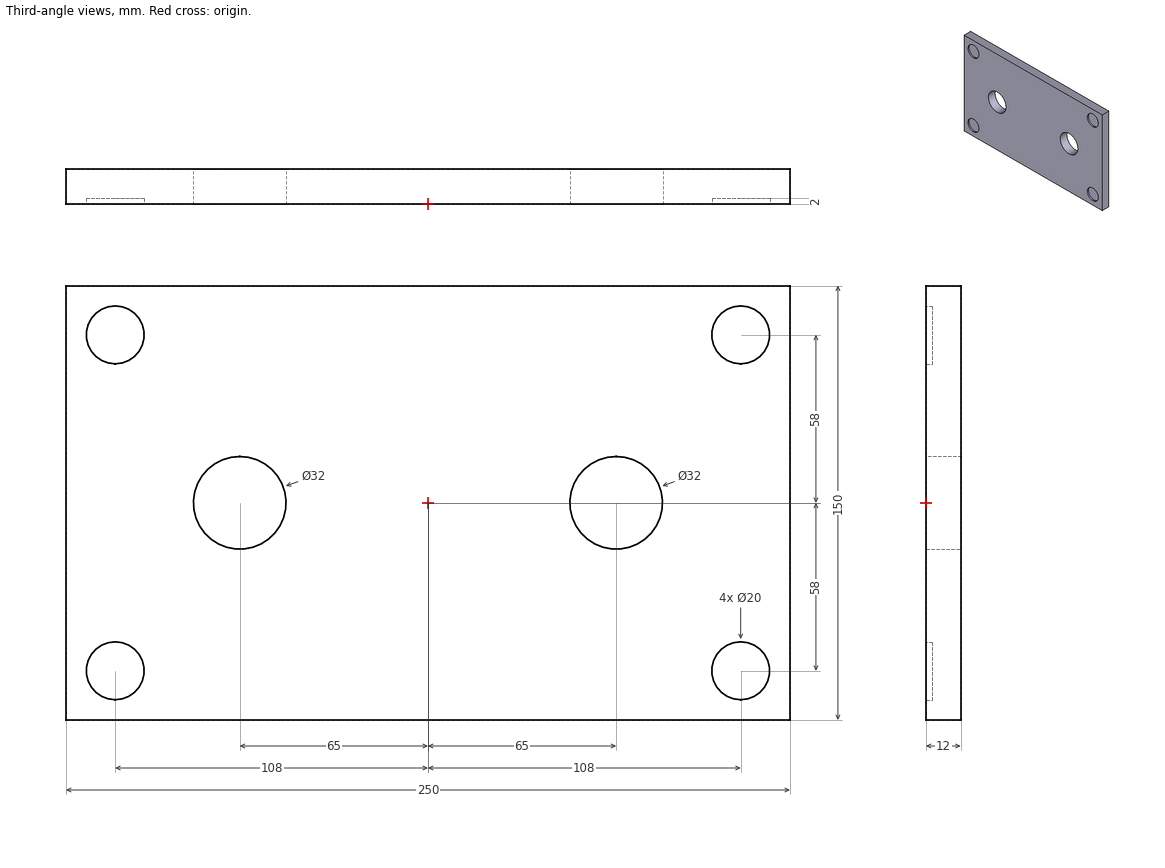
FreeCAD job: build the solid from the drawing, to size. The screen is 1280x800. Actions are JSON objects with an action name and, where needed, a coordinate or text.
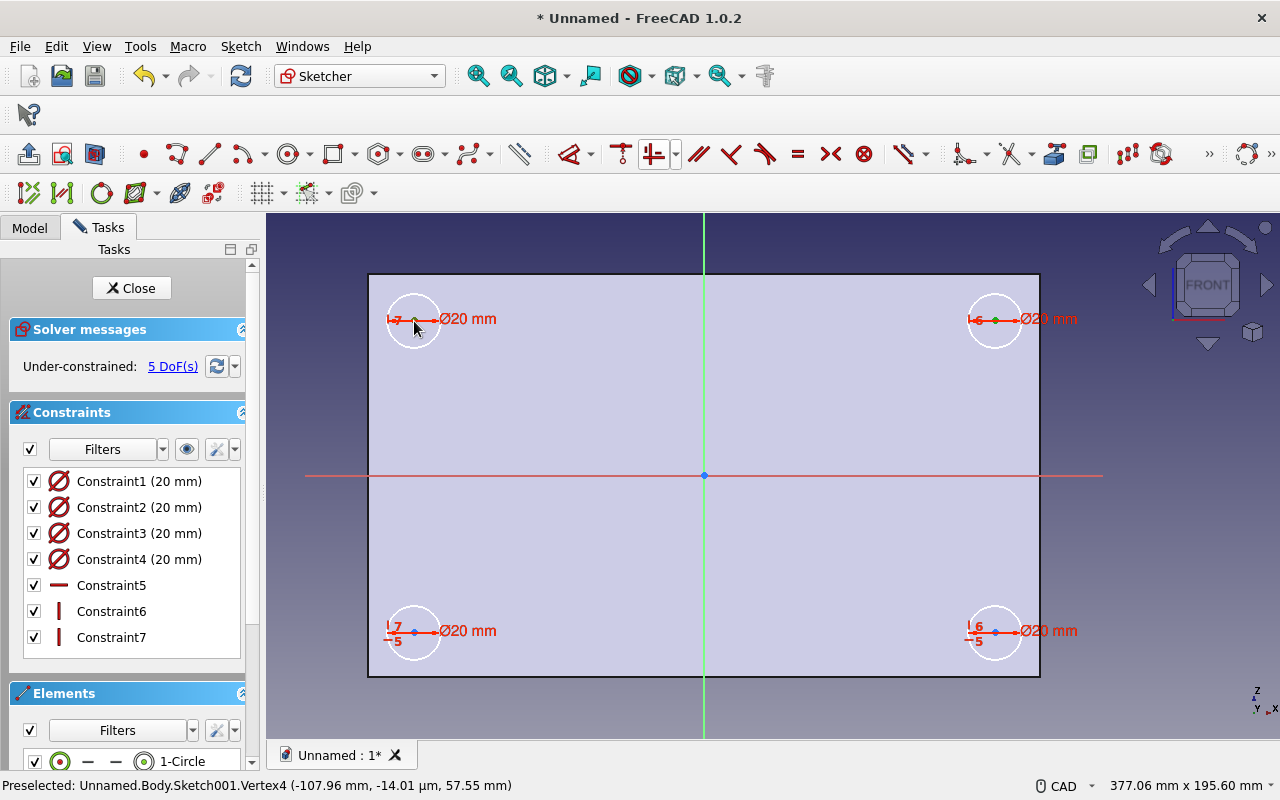
{"action": "left_click", "coordinate": [676, 154]}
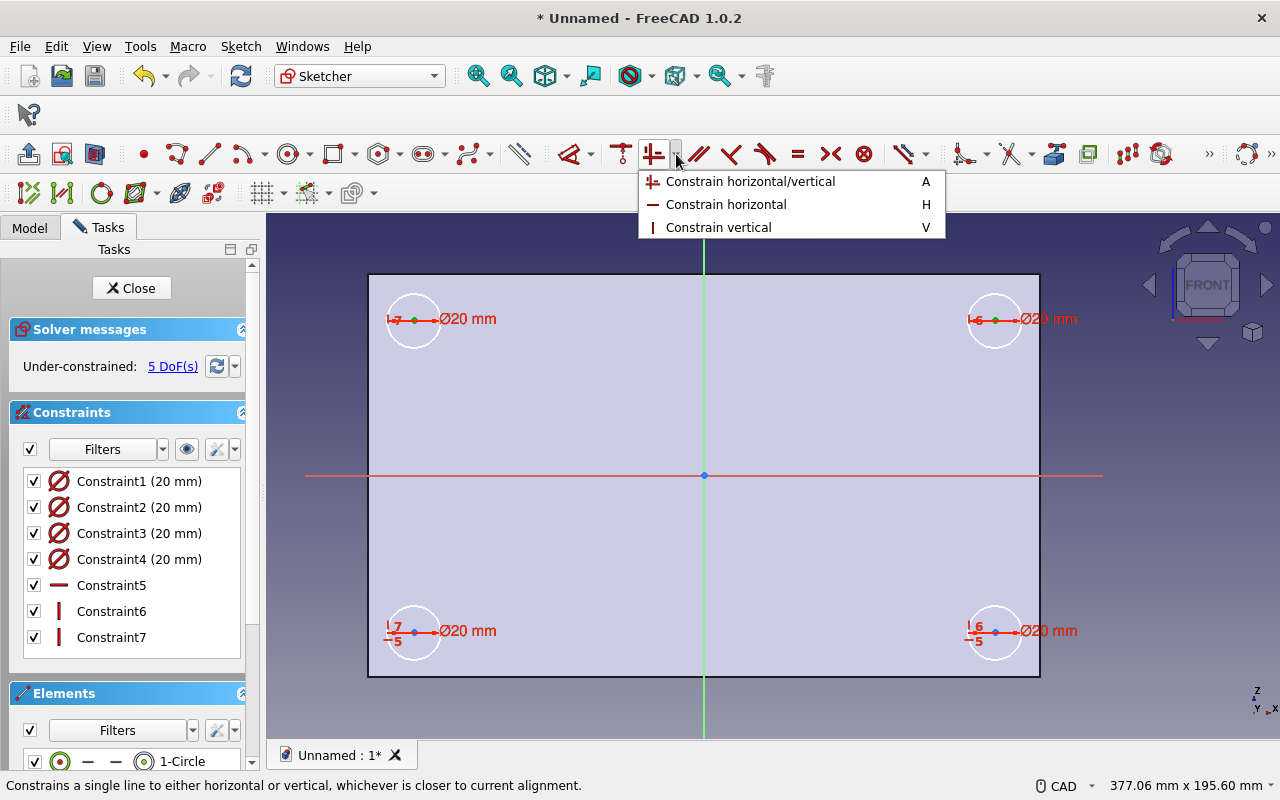
{"action": "left_click", "coordinate": [792, 204]}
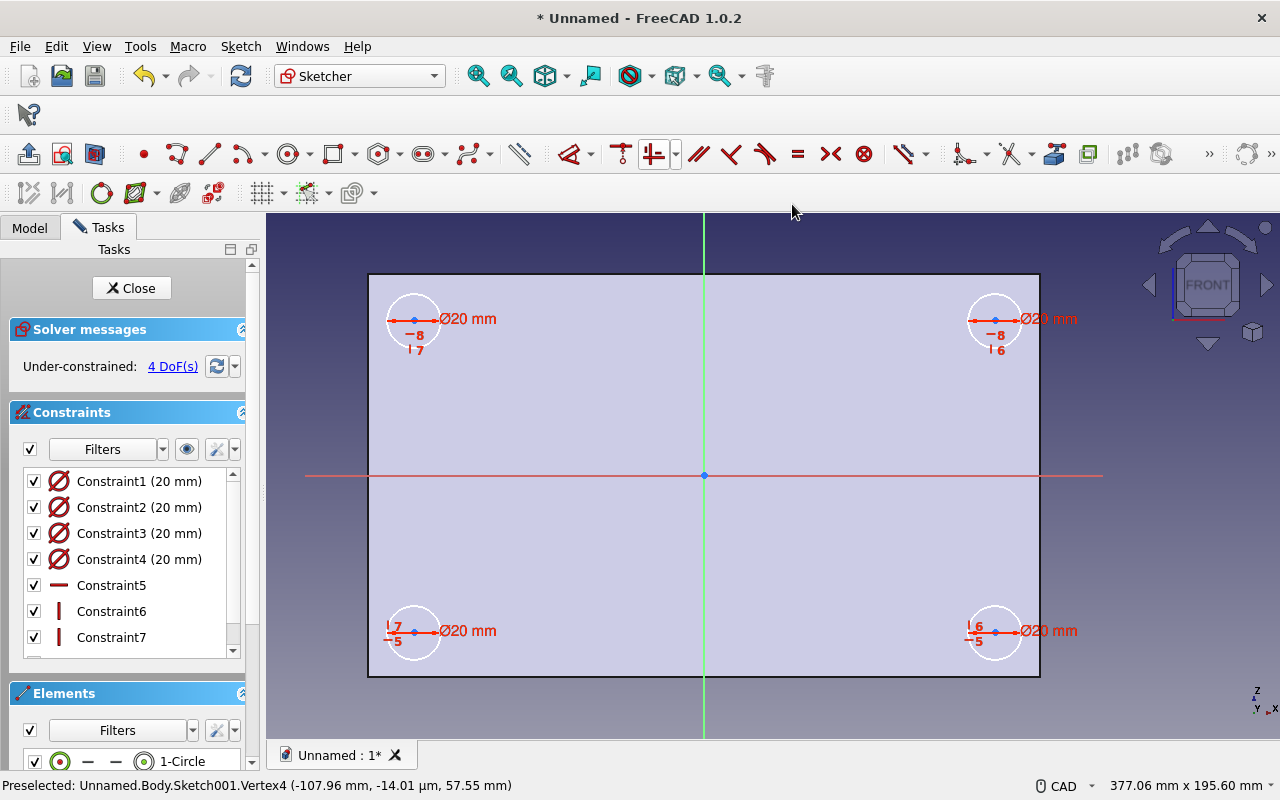
{"action": "left_click", "coordinate": [568, 154]}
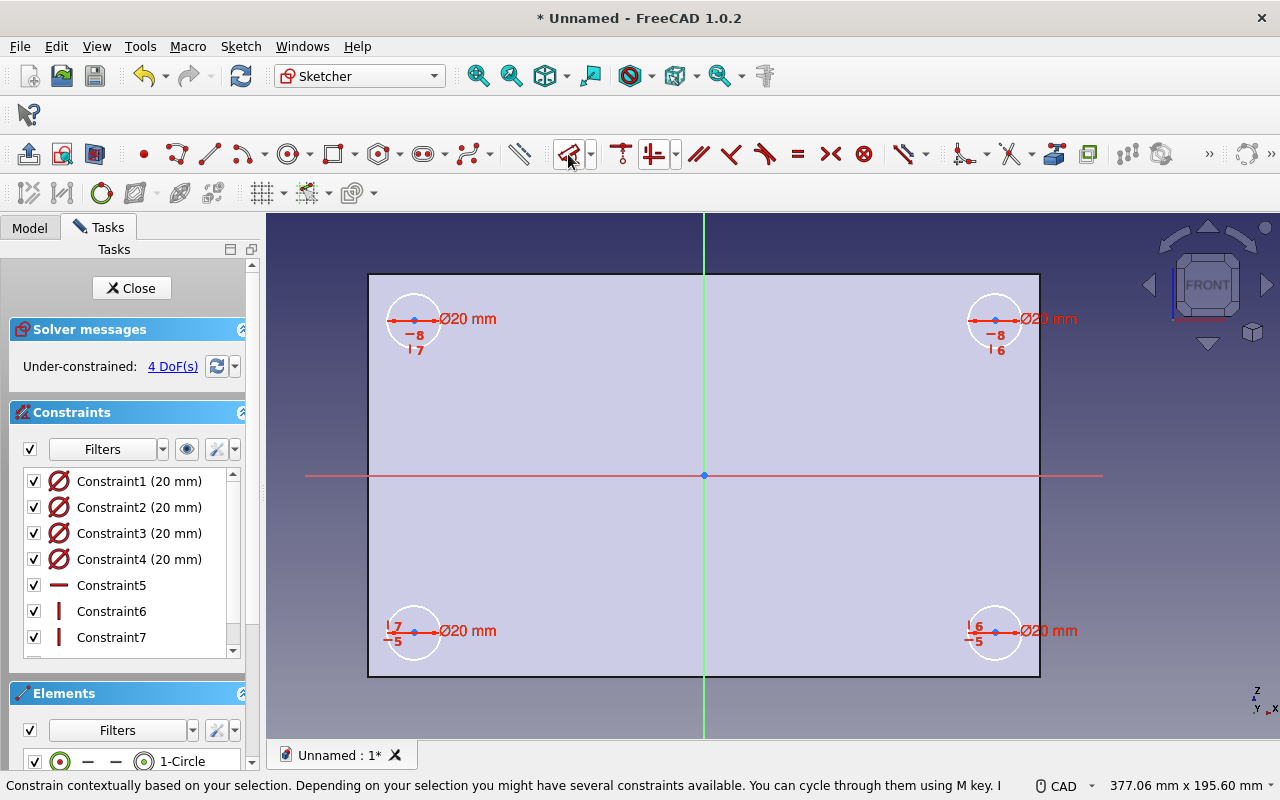
{"action": "left_click", "coordinate": [995, 633]}
{"action": "left_click", "coordinate": [1029, 554]}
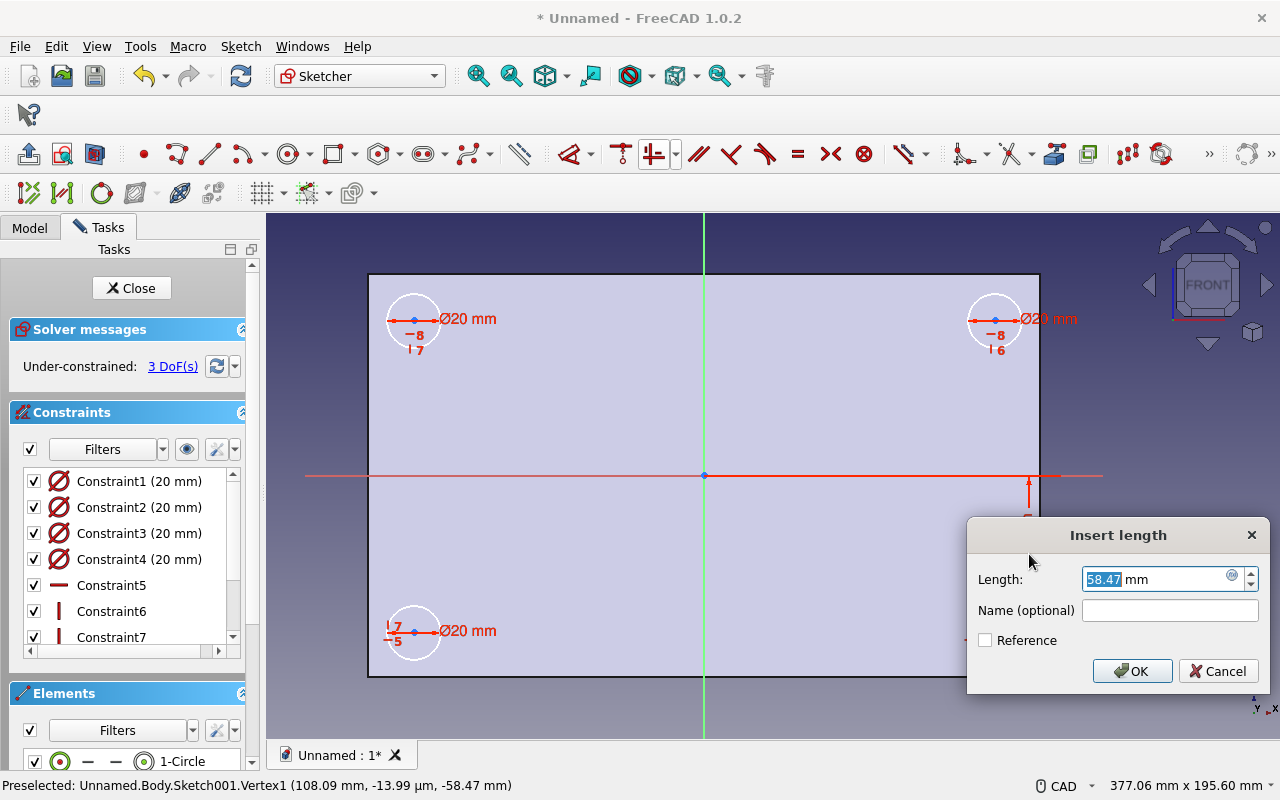
{"action": "type", "text": "58"}
{"action": "key", "text": "Return"}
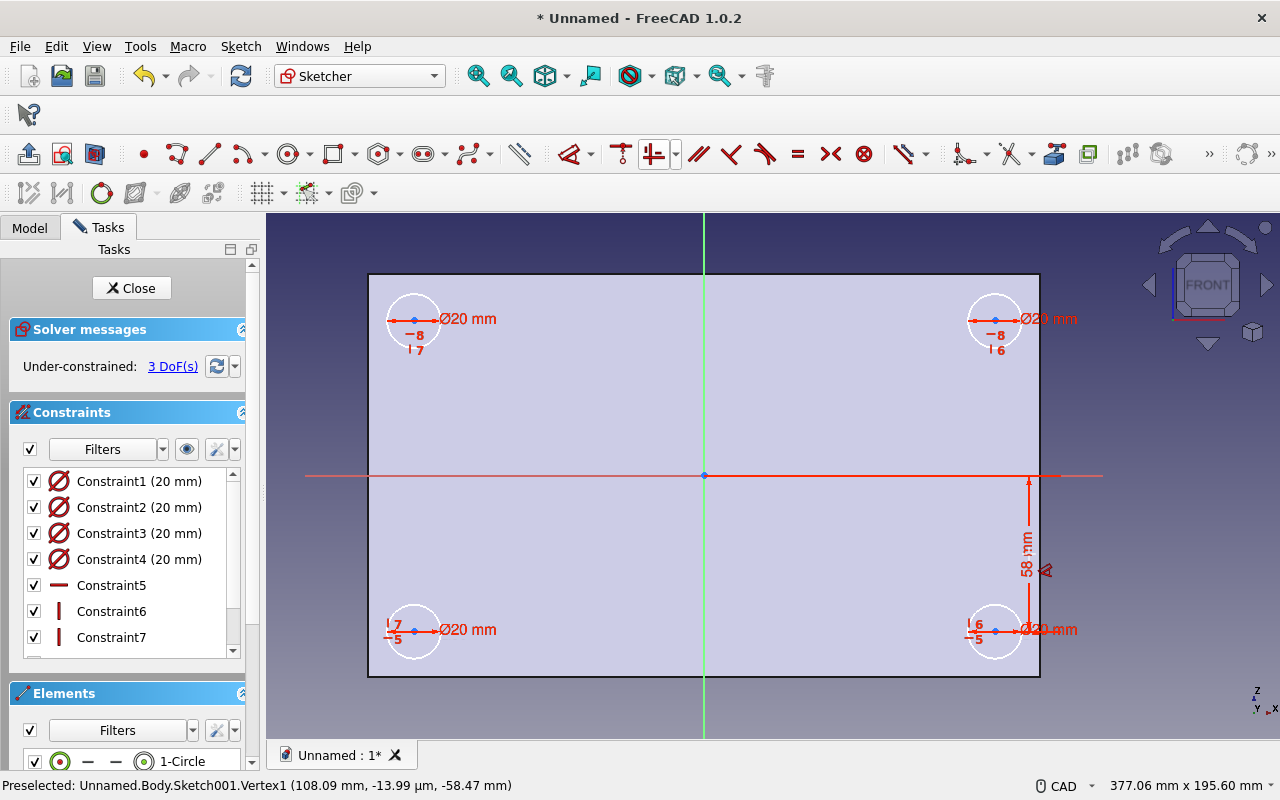
{"action": "left_click", "coordinate": [995, 321]}
{"action": "left_click", "coordinate": [1029, 398]}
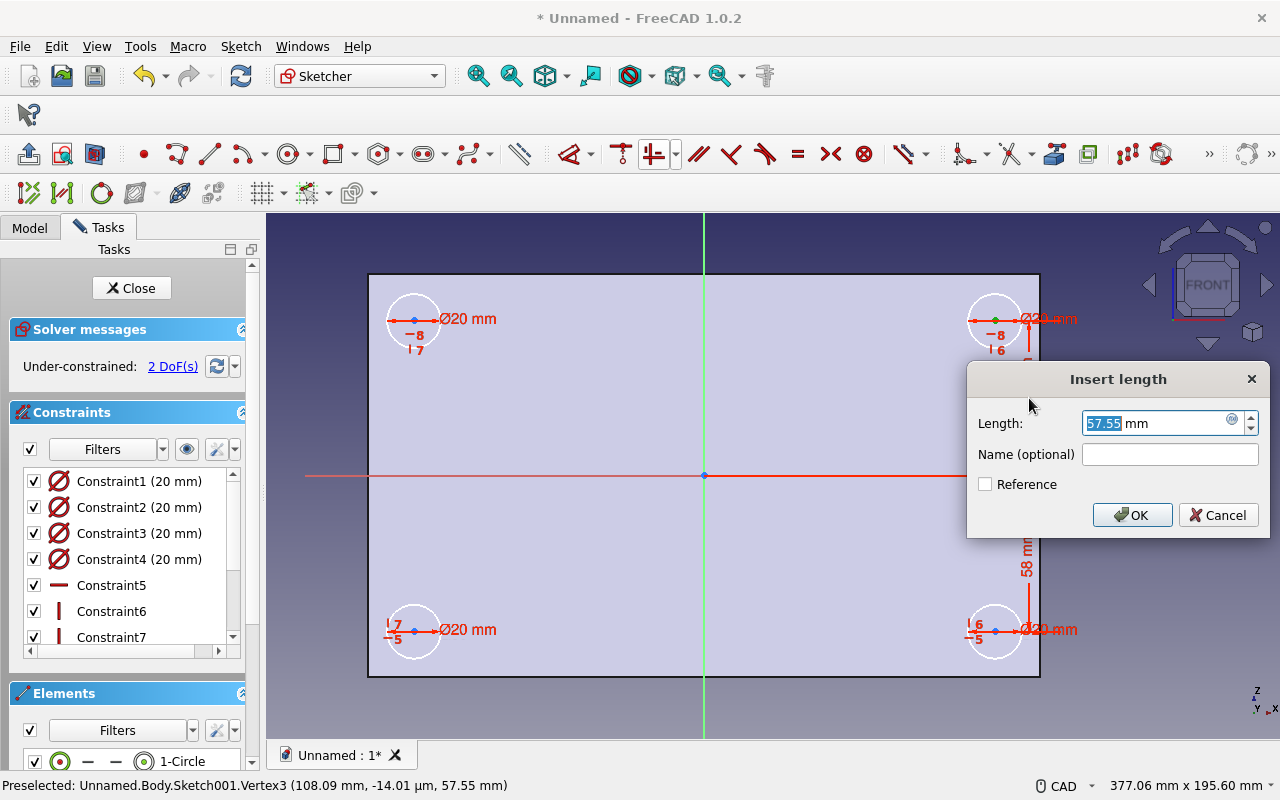
{"action": "type", "text": "58"}
{"action": "key", "text": "Return"}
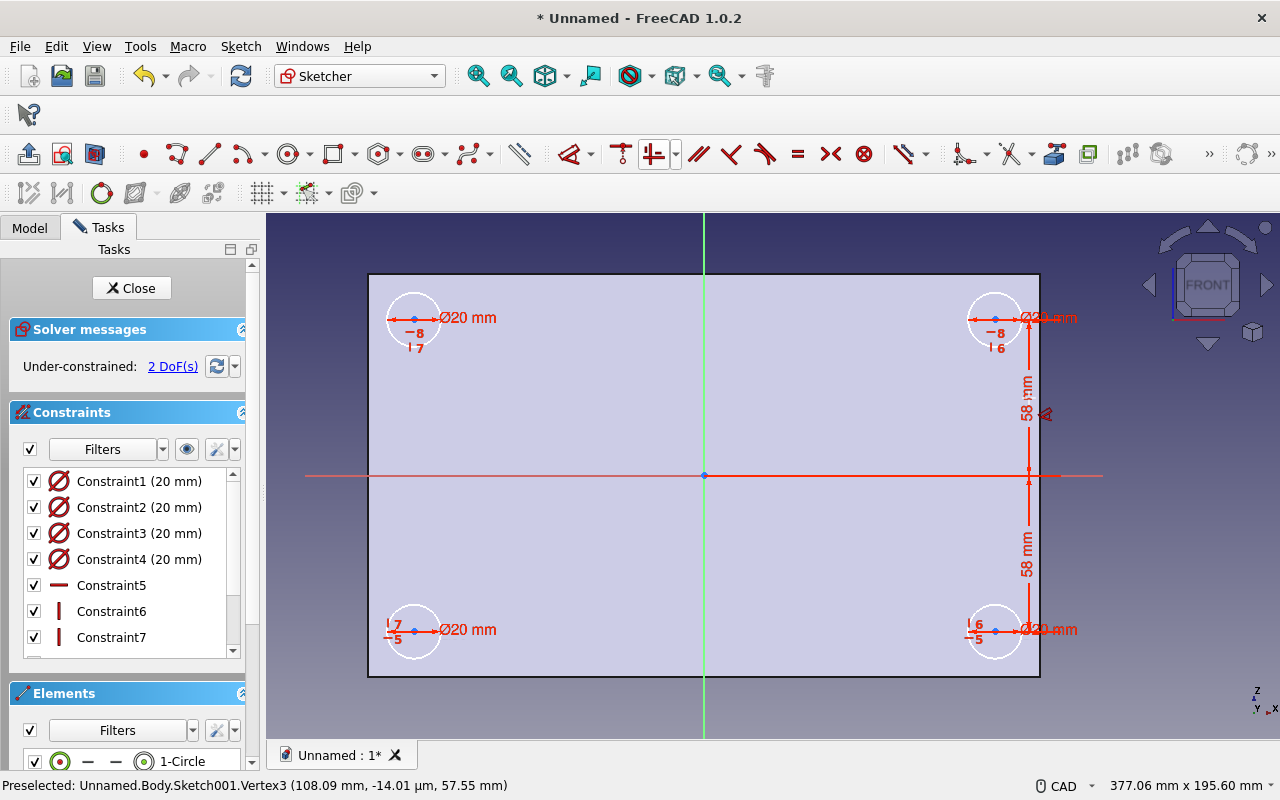
{"action": "left_click", "coordinate": [995, 632]}
{"action": "left_click", "coordinate": [850, 666]}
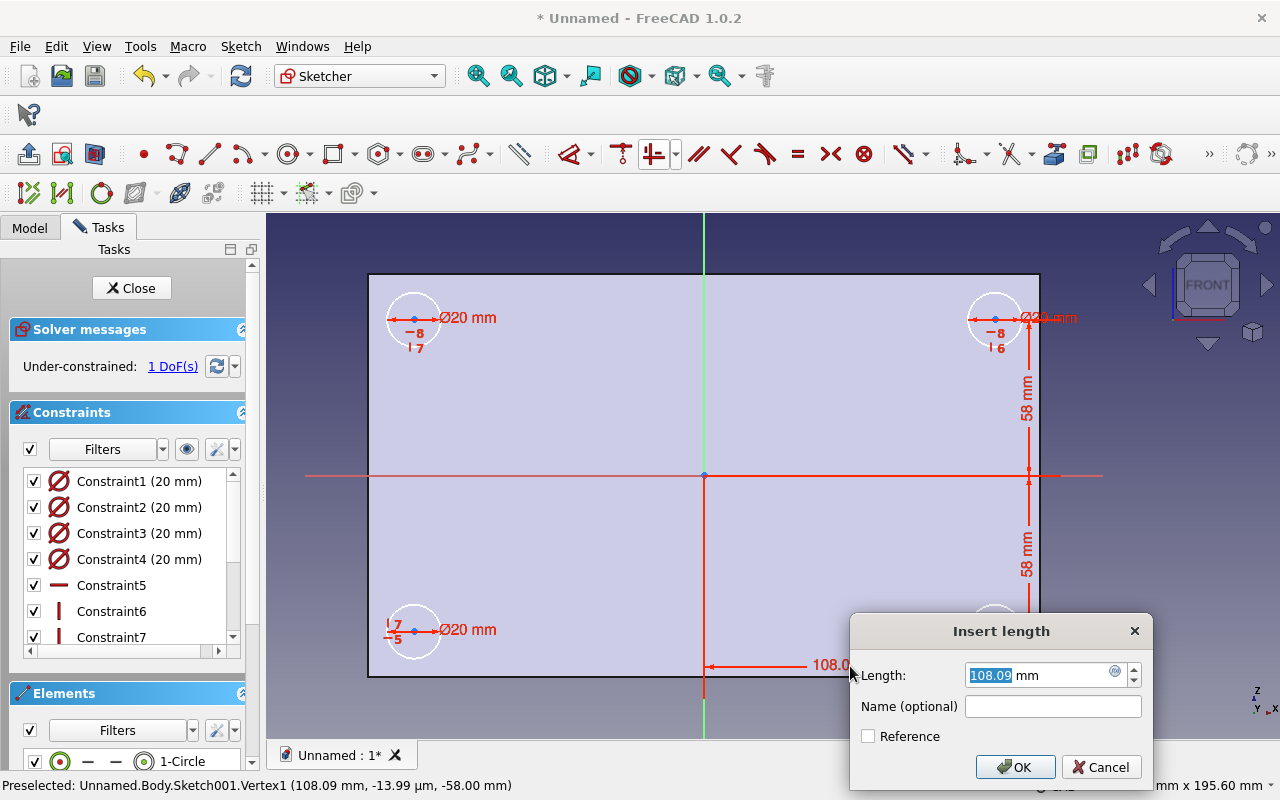
{"action": "type", "text": "108"}
{"action": "key", "text": "Return"}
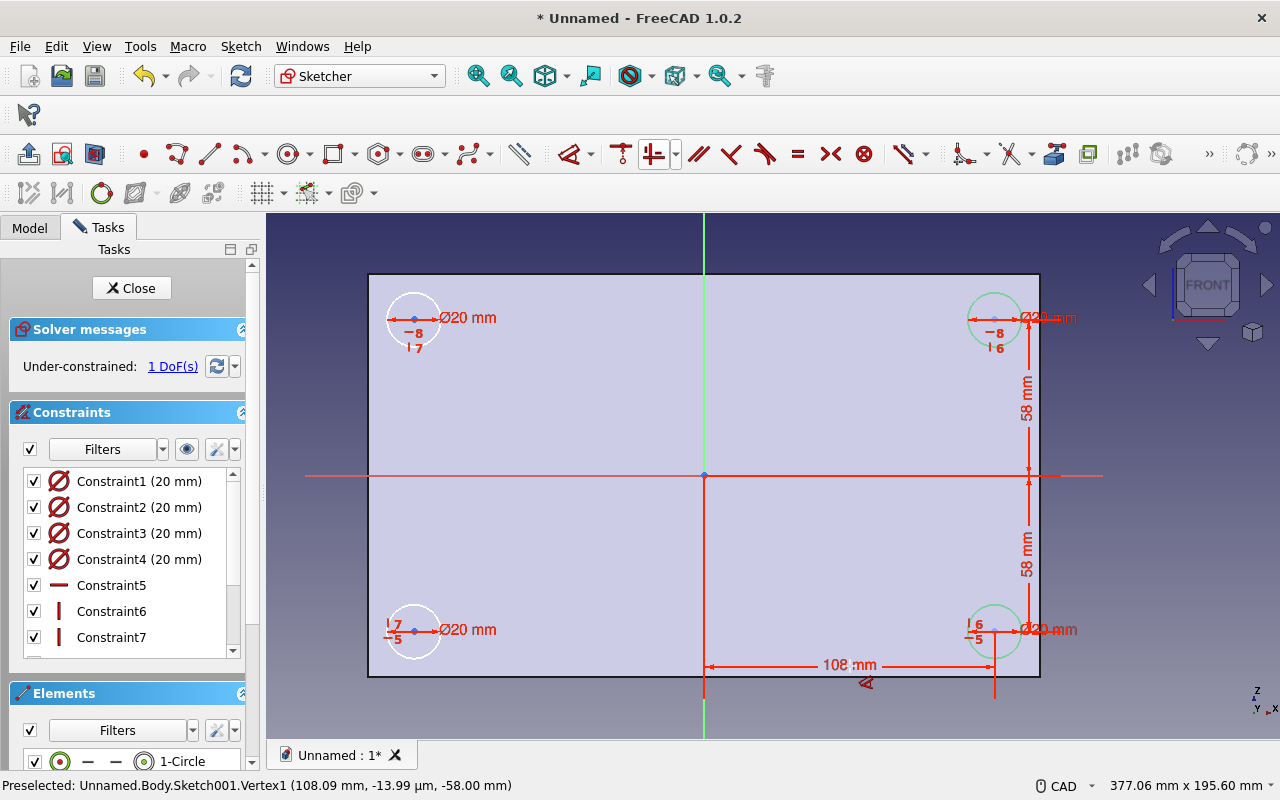
{"action": "left_click", "coordinate": [414, 632]}
{"action": "left_click", "coordinate": [559, 666]}